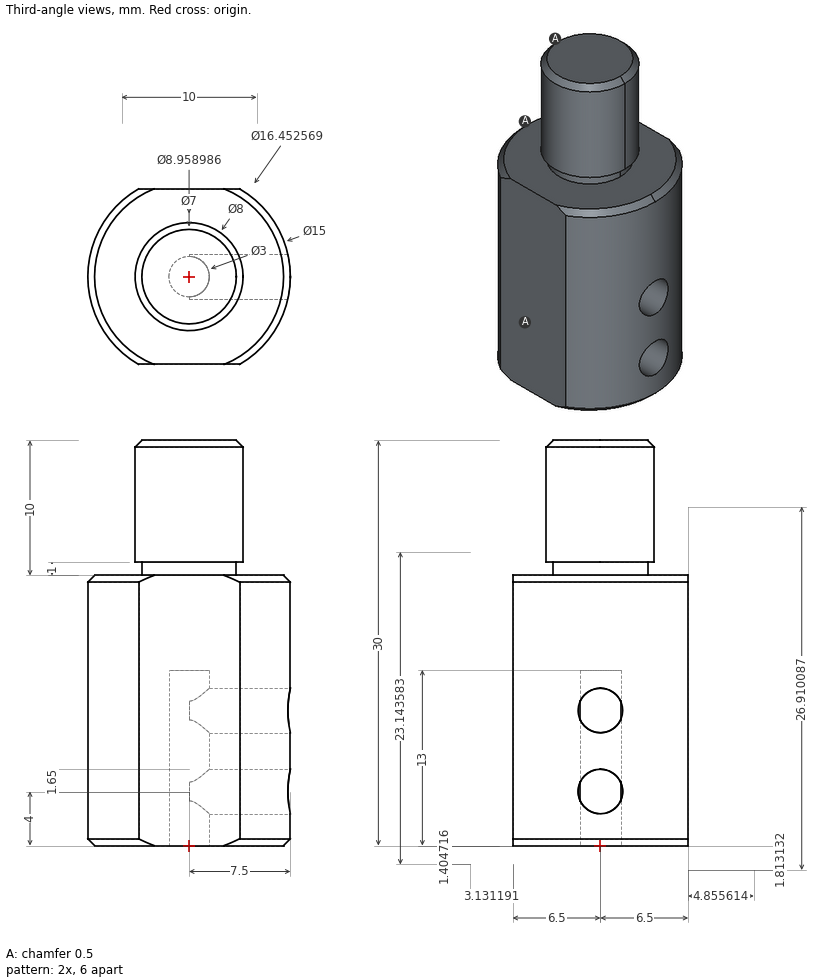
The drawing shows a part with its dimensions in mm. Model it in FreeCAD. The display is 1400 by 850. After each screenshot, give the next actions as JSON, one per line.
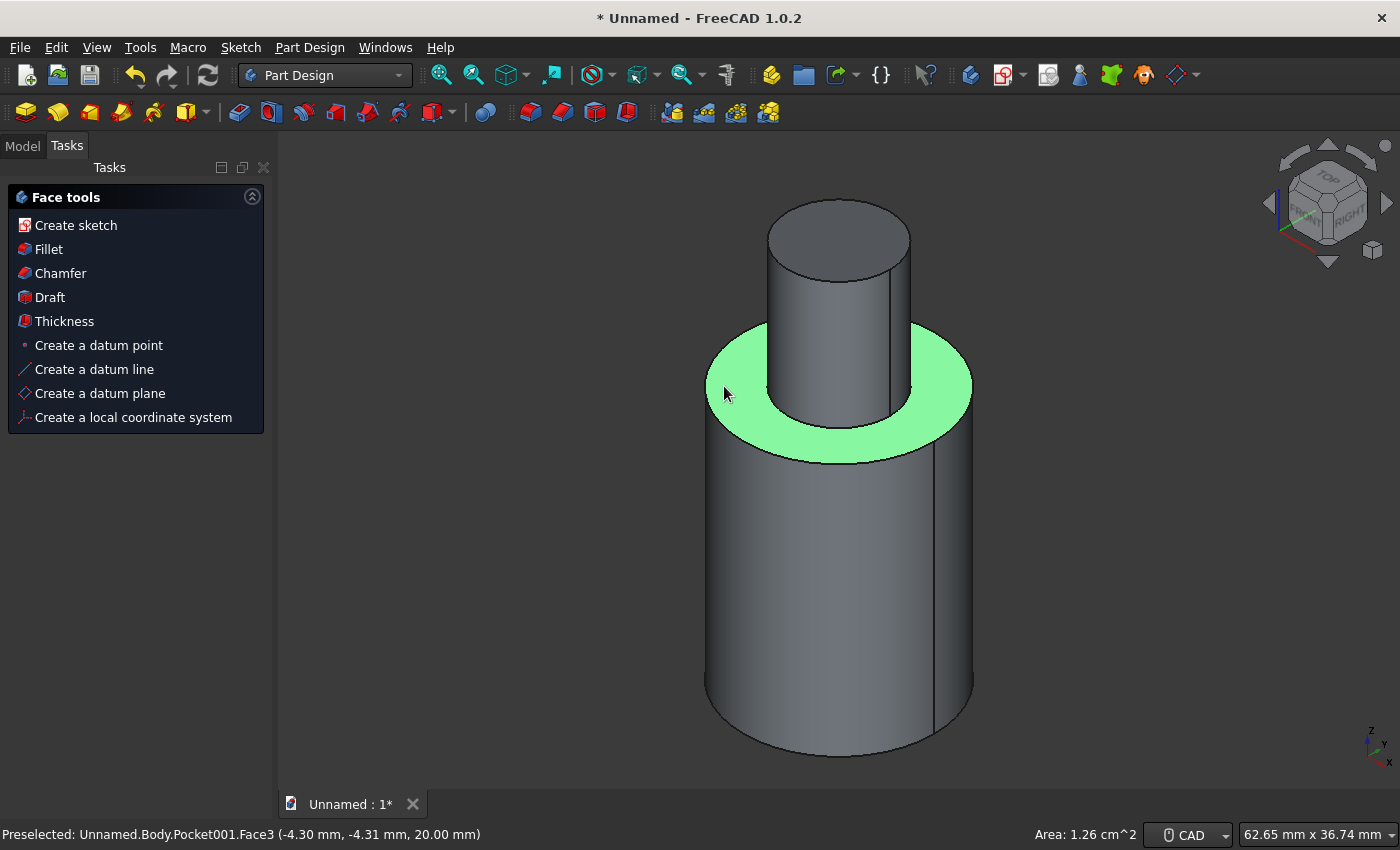
{"action": "left_click", "coordinate": [1004, 76]}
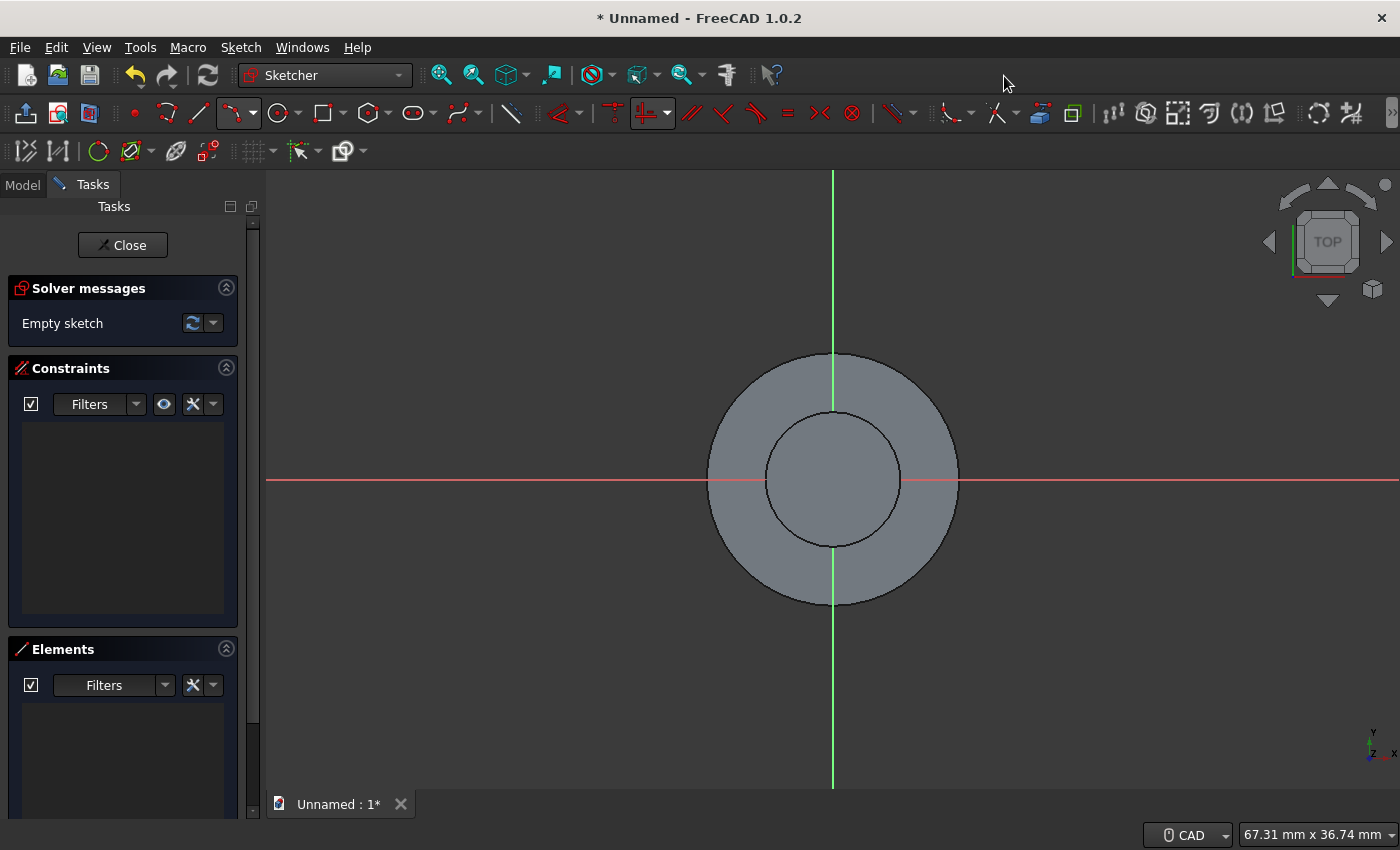
{"action": "scroll", "coordinate": [873, 480], "scroll_direction": "up", "scroll_amount": 5}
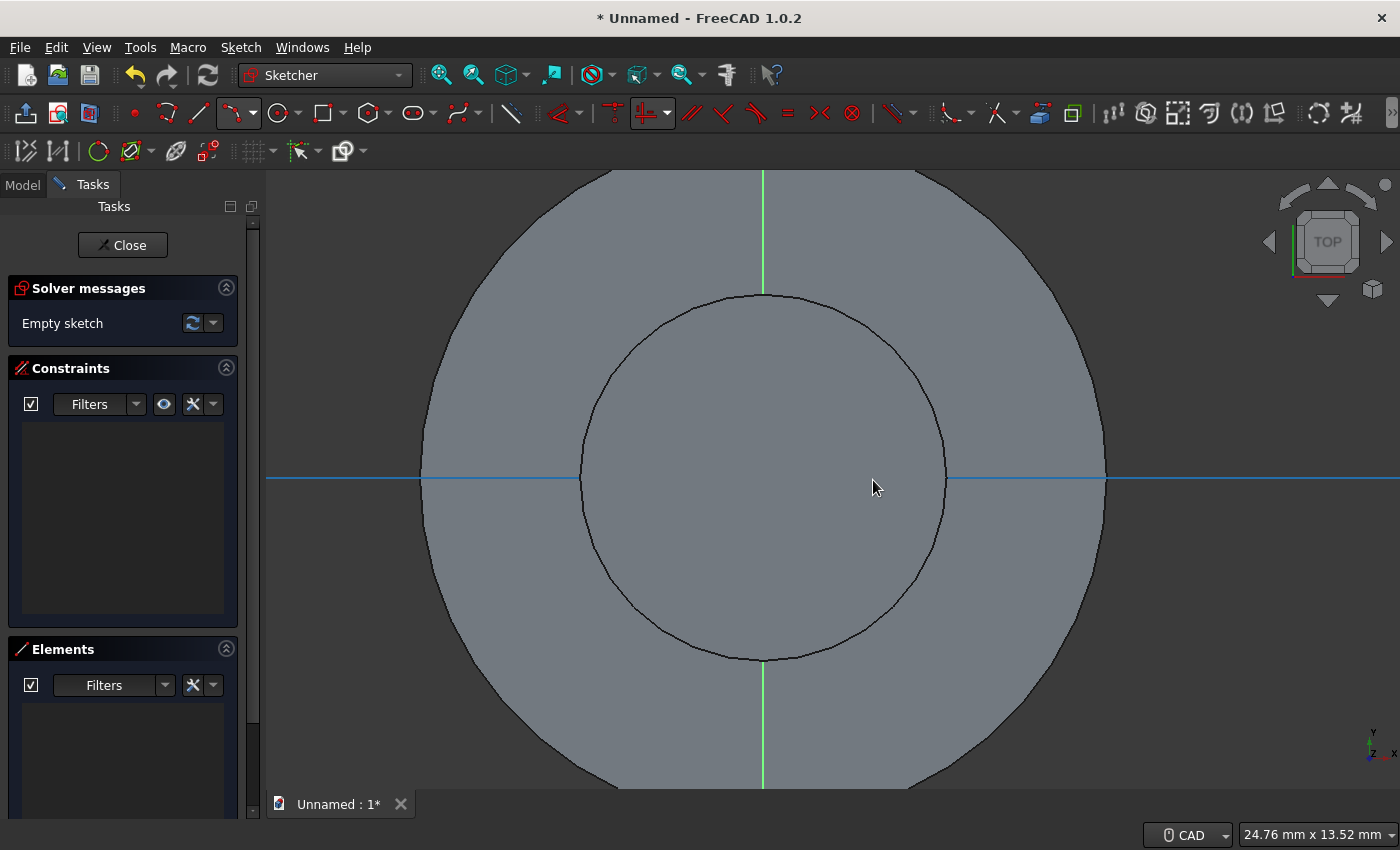
{"action": "left_click", "coordinate": [278, 114]}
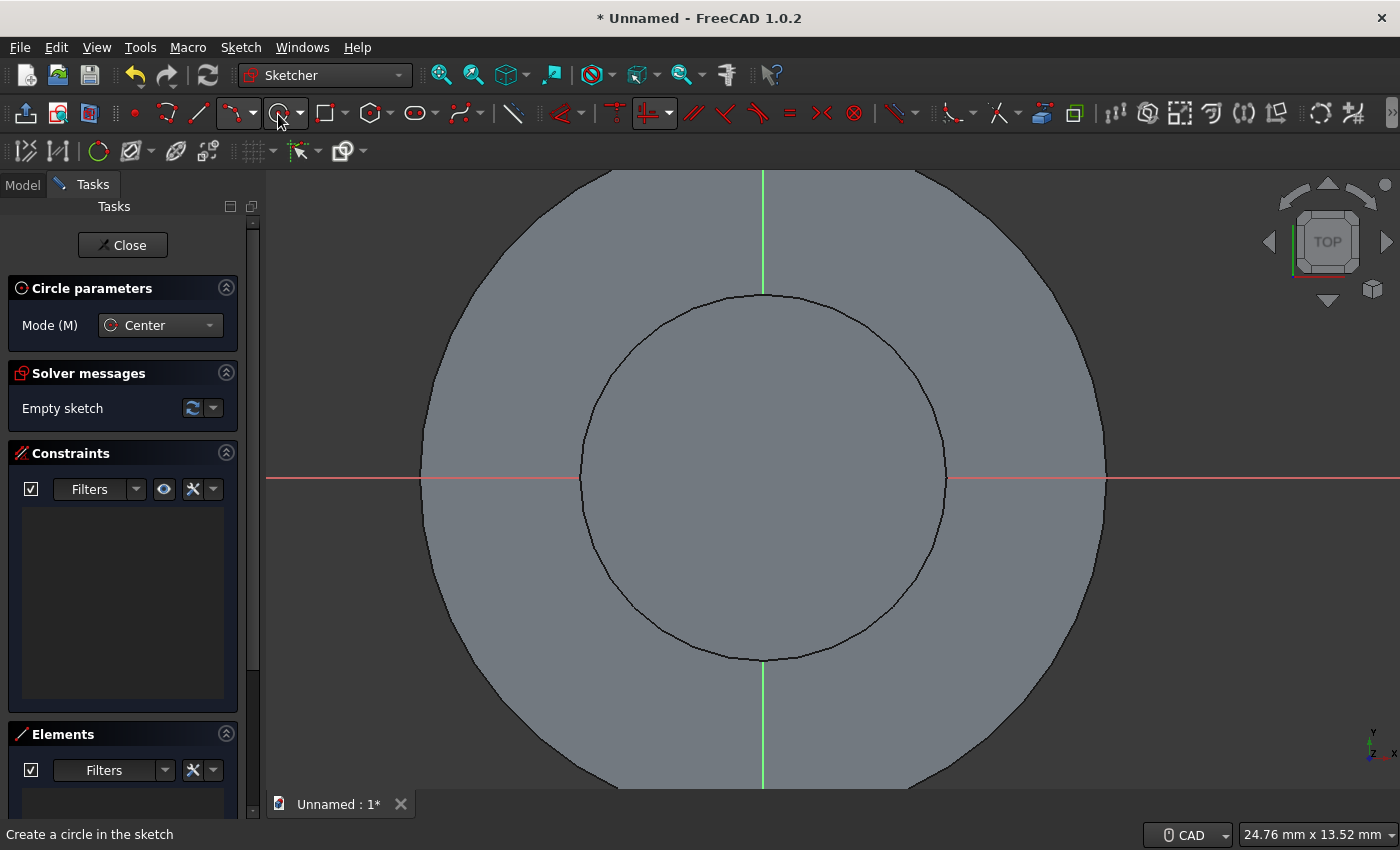
{"action": "left_click", "coordinate": [763, 478]}
{"action": "left_click", "coordinate": [908, 333]}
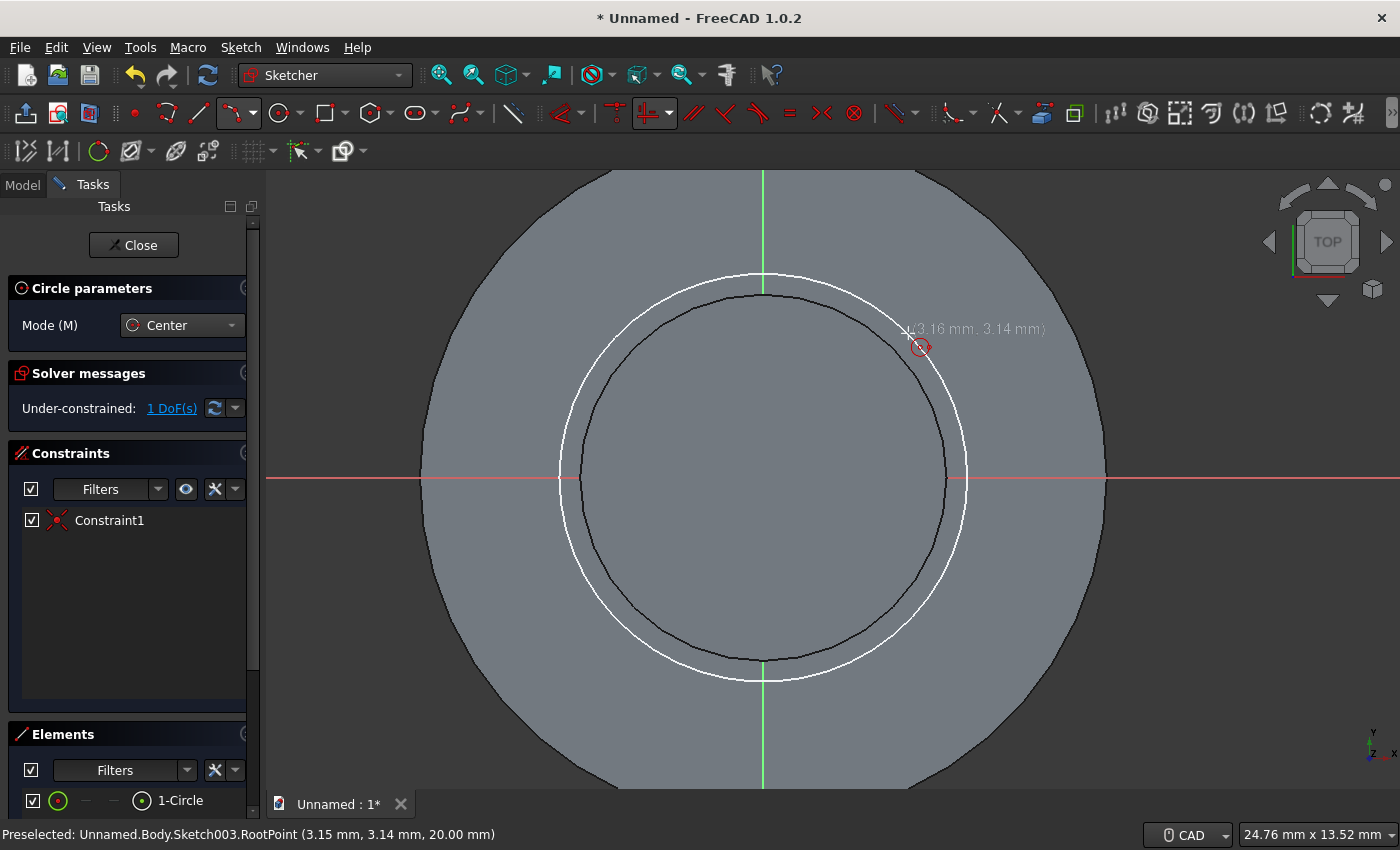
{"action": "left_click", "coordinate": [763, 478]}
{"action": "left_click", "coordinate": [877, 364]}
{"action": "key", "text": "Escape"}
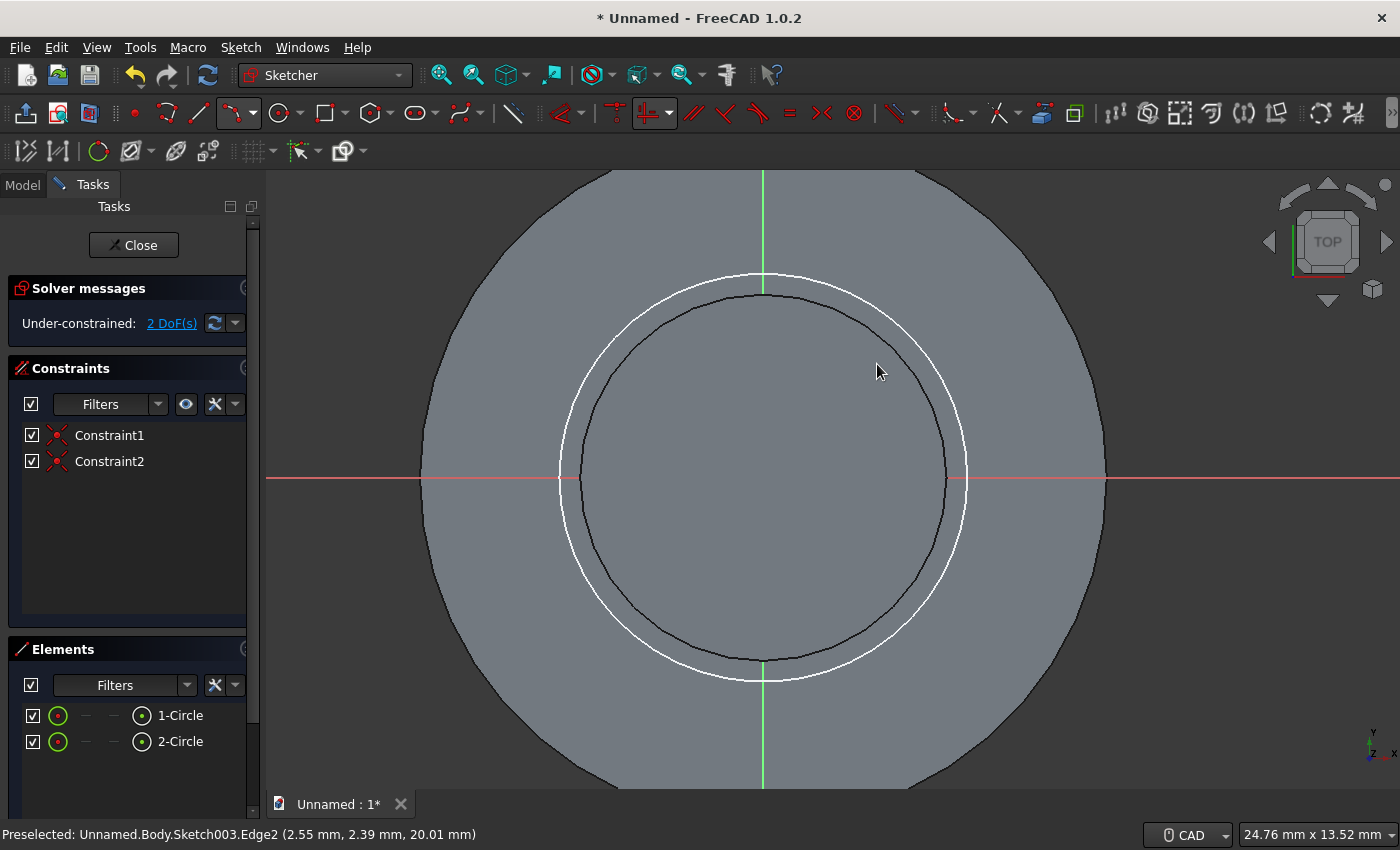
{"action": "left_click", "coordinate": [560, 114]}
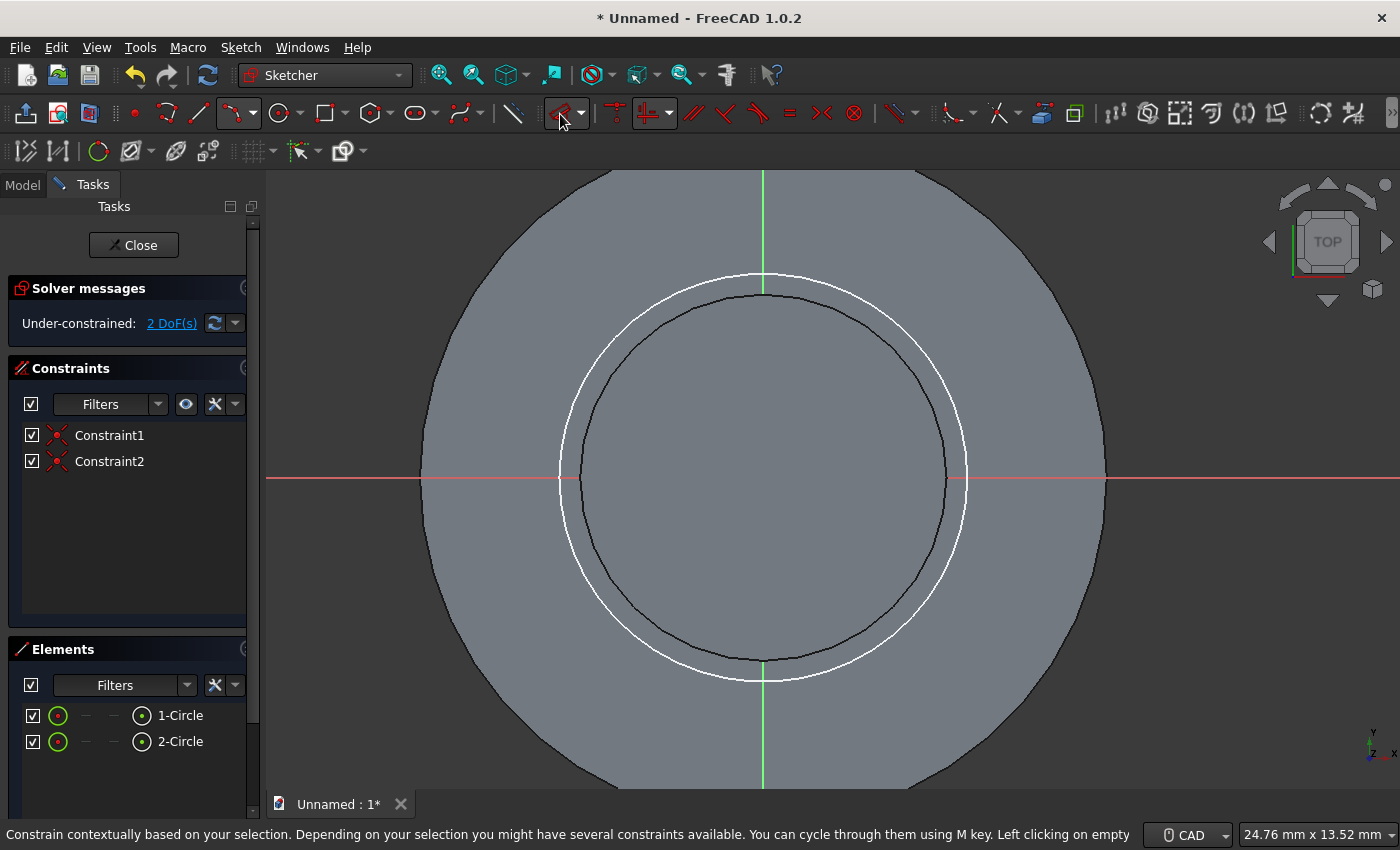
{"action": "left_click", "coordinate": [907, 333]}
{"action": "left_click", "coordinate": [930, 310]}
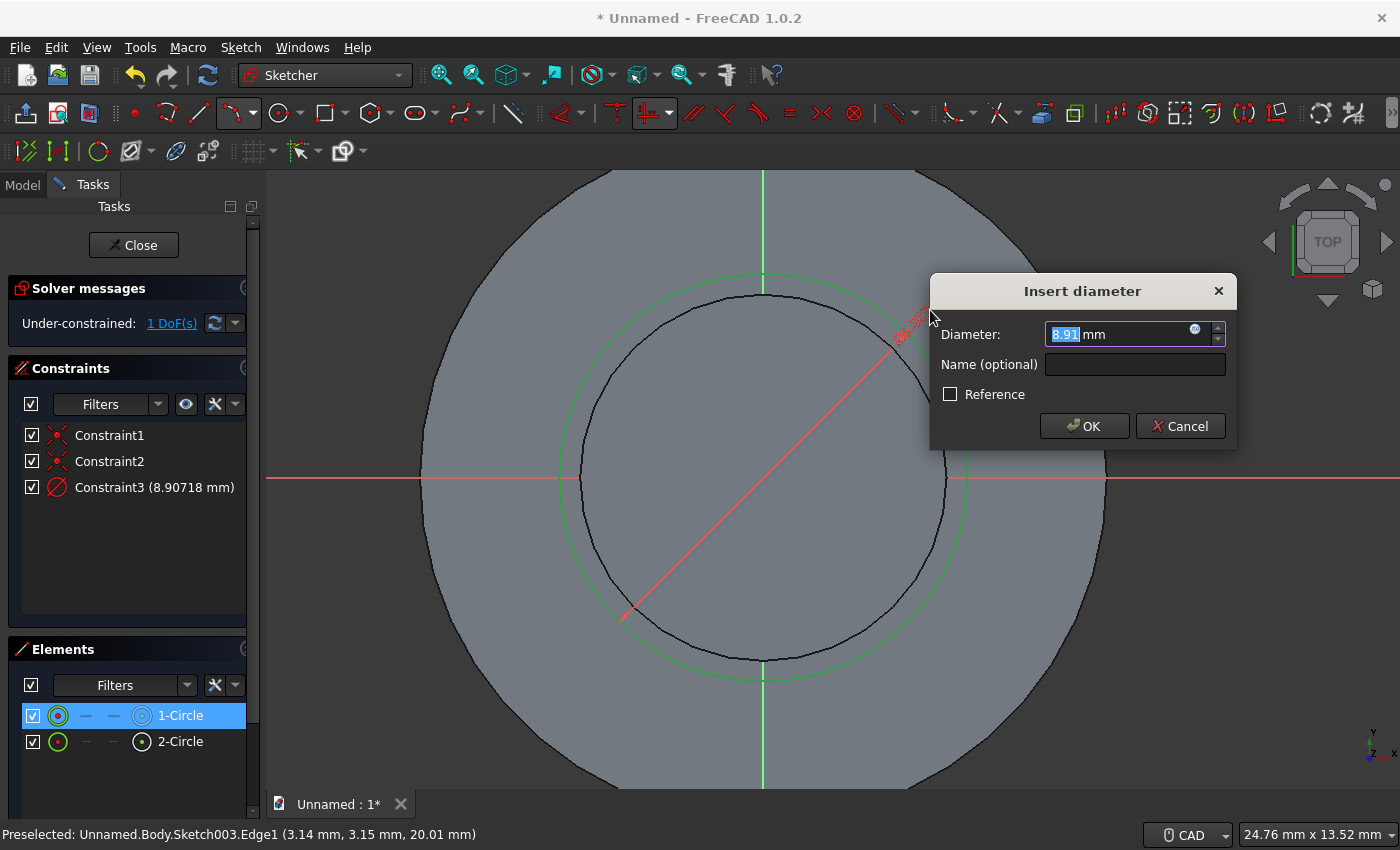
{"action": "type", "text": "8.958986"}
{"action": "key", "text": "Return"}